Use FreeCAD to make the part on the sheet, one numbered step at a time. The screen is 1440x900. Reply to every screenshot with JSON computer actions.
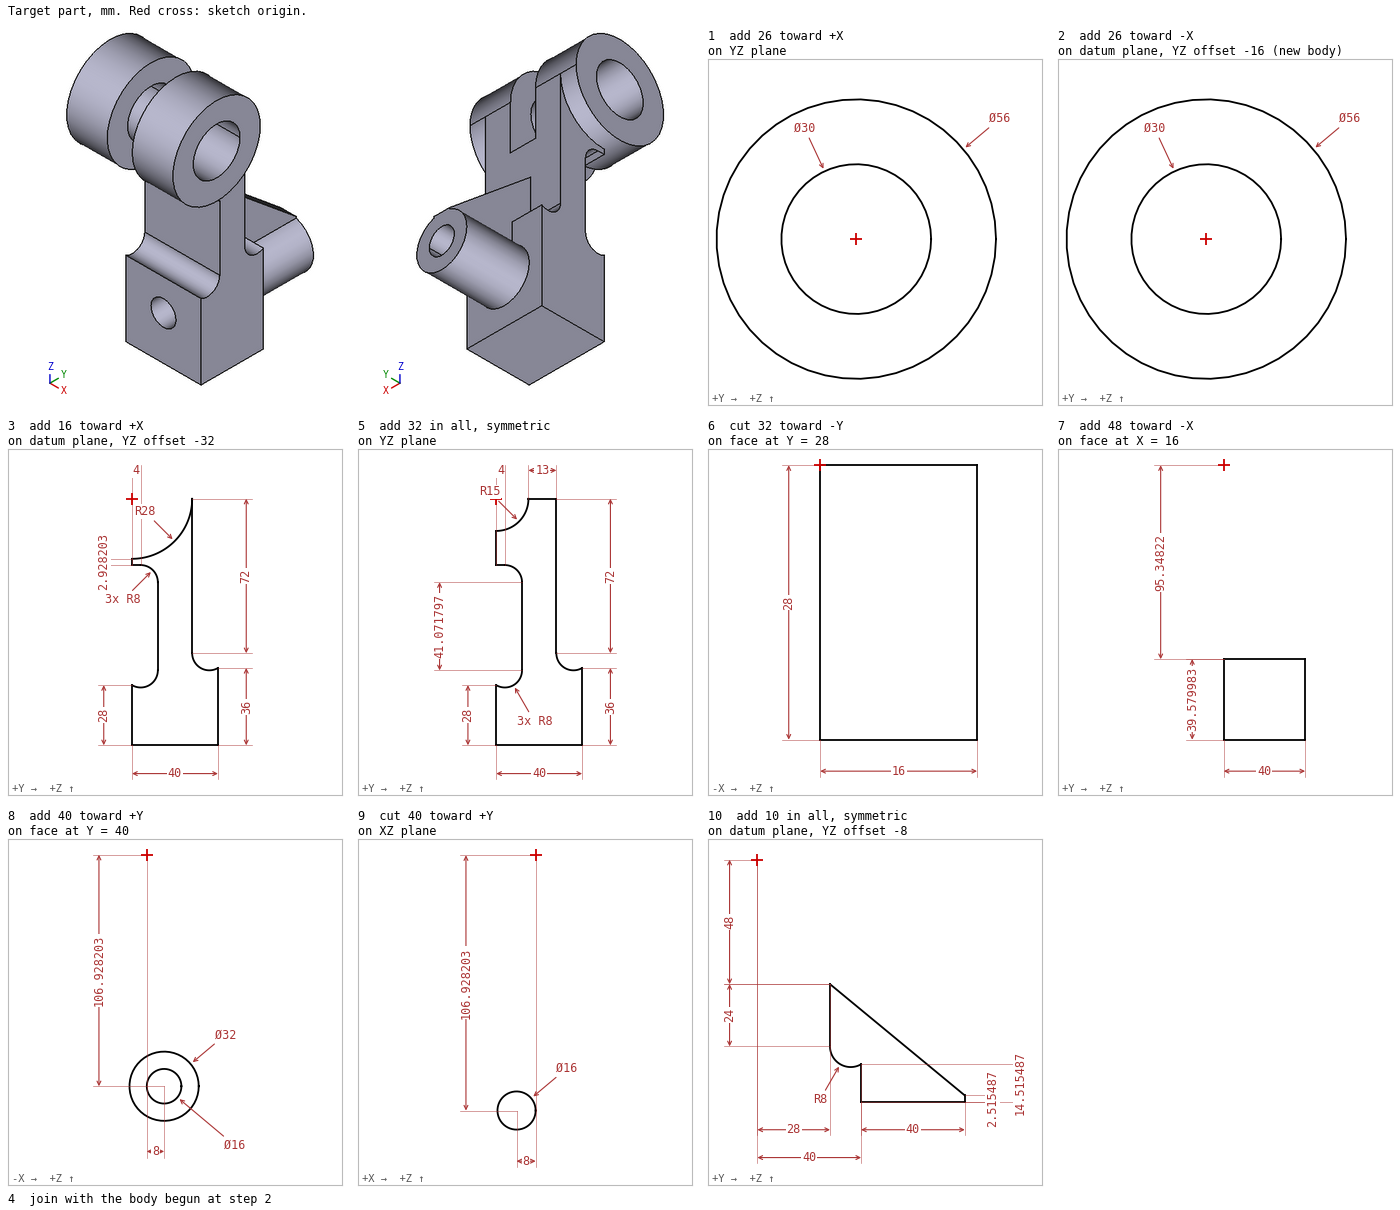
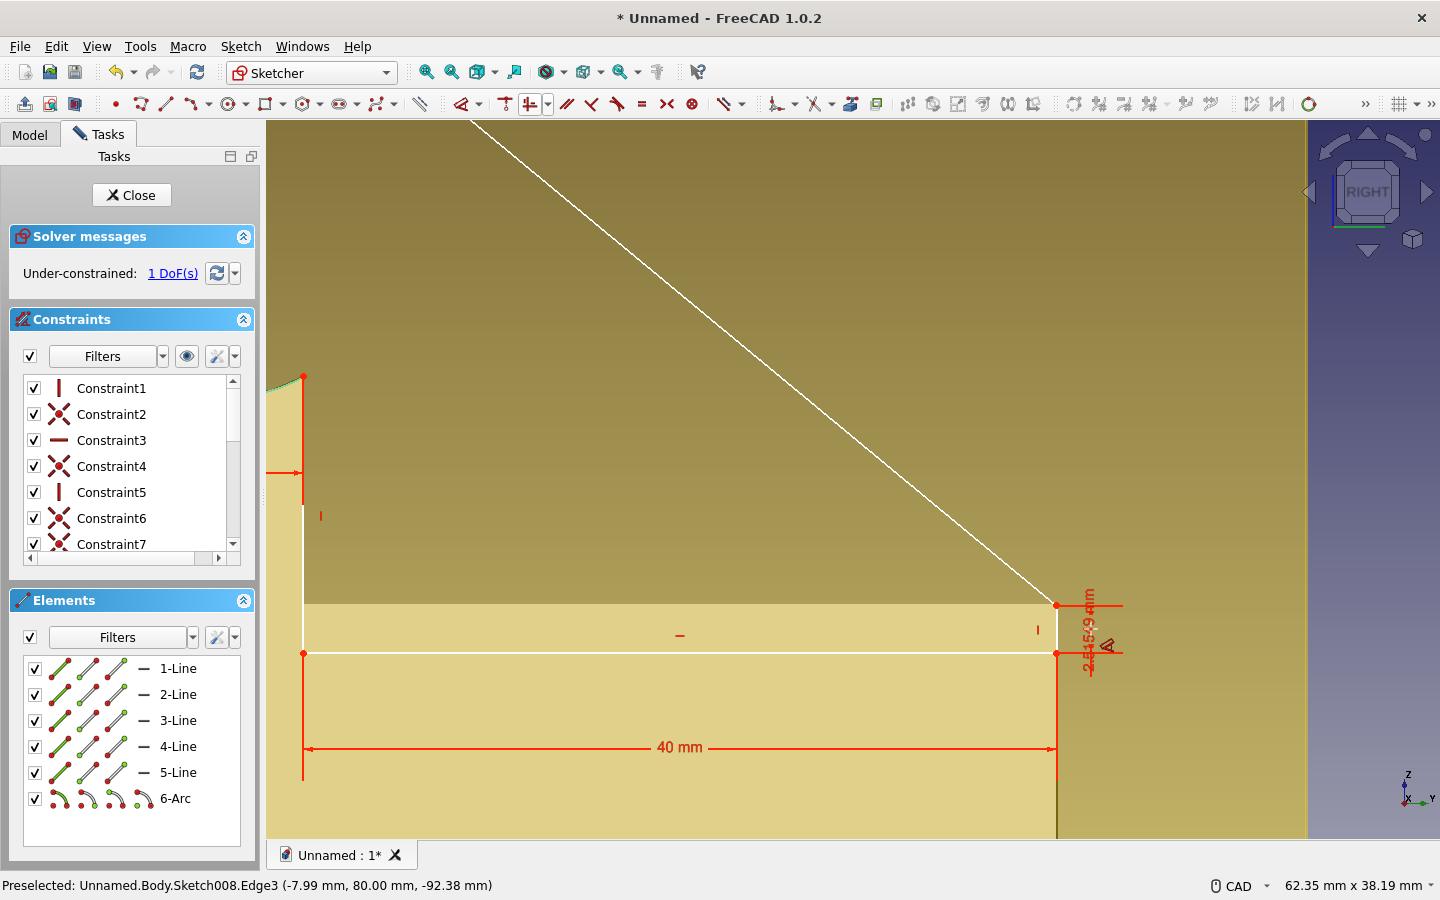
{"action": "scroll", "coordinate": [942, 712], "scroll_direction": "down", "scroll_amount": 7}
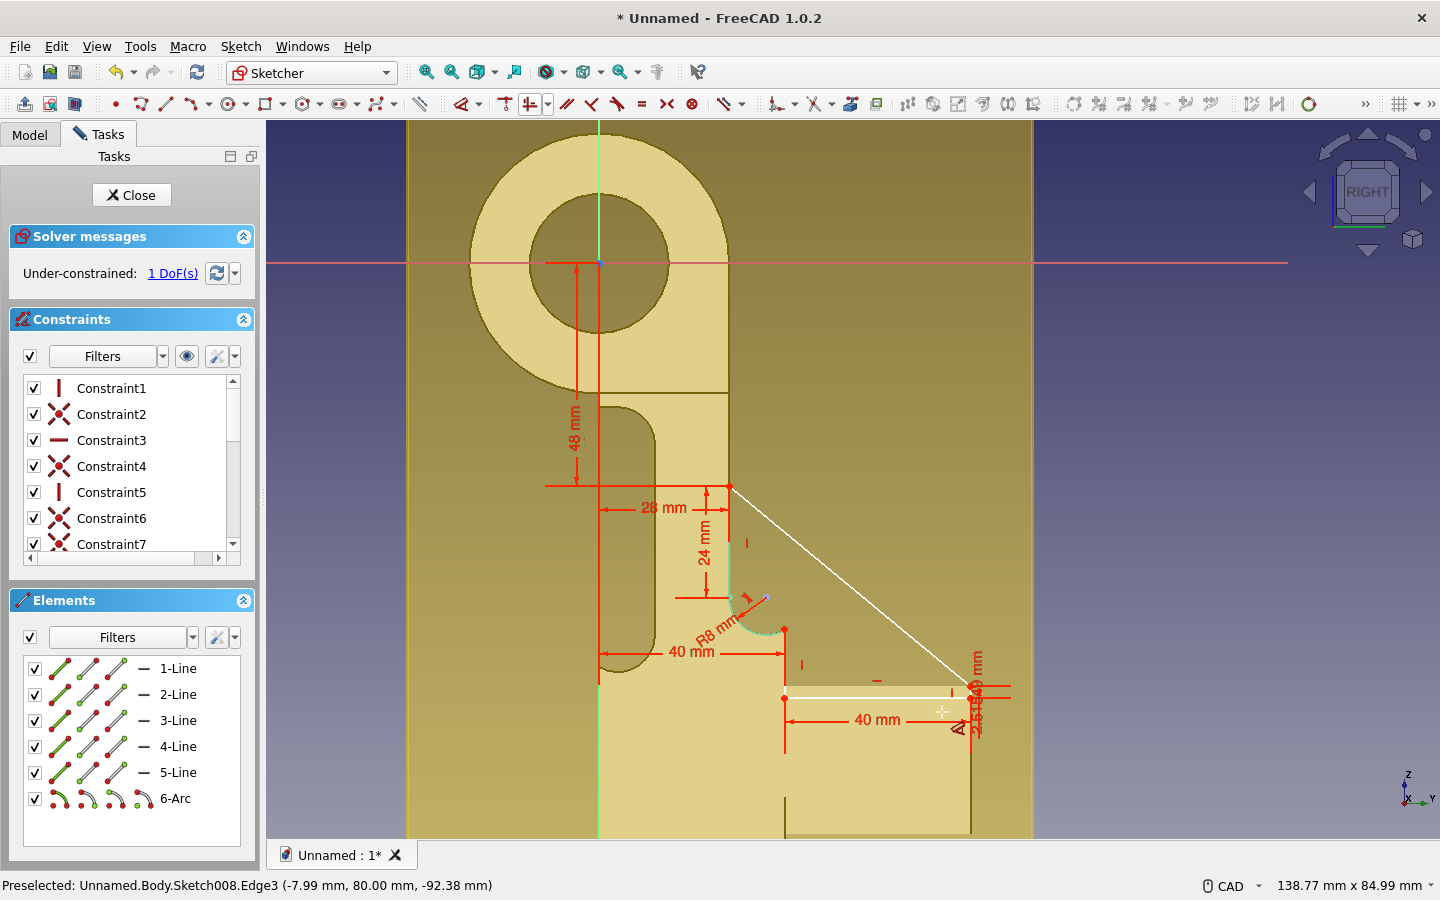
{"action": "left_click", "coordinate": [785, 650]}
{"action": "left_click", "coordinate": [819, 664]}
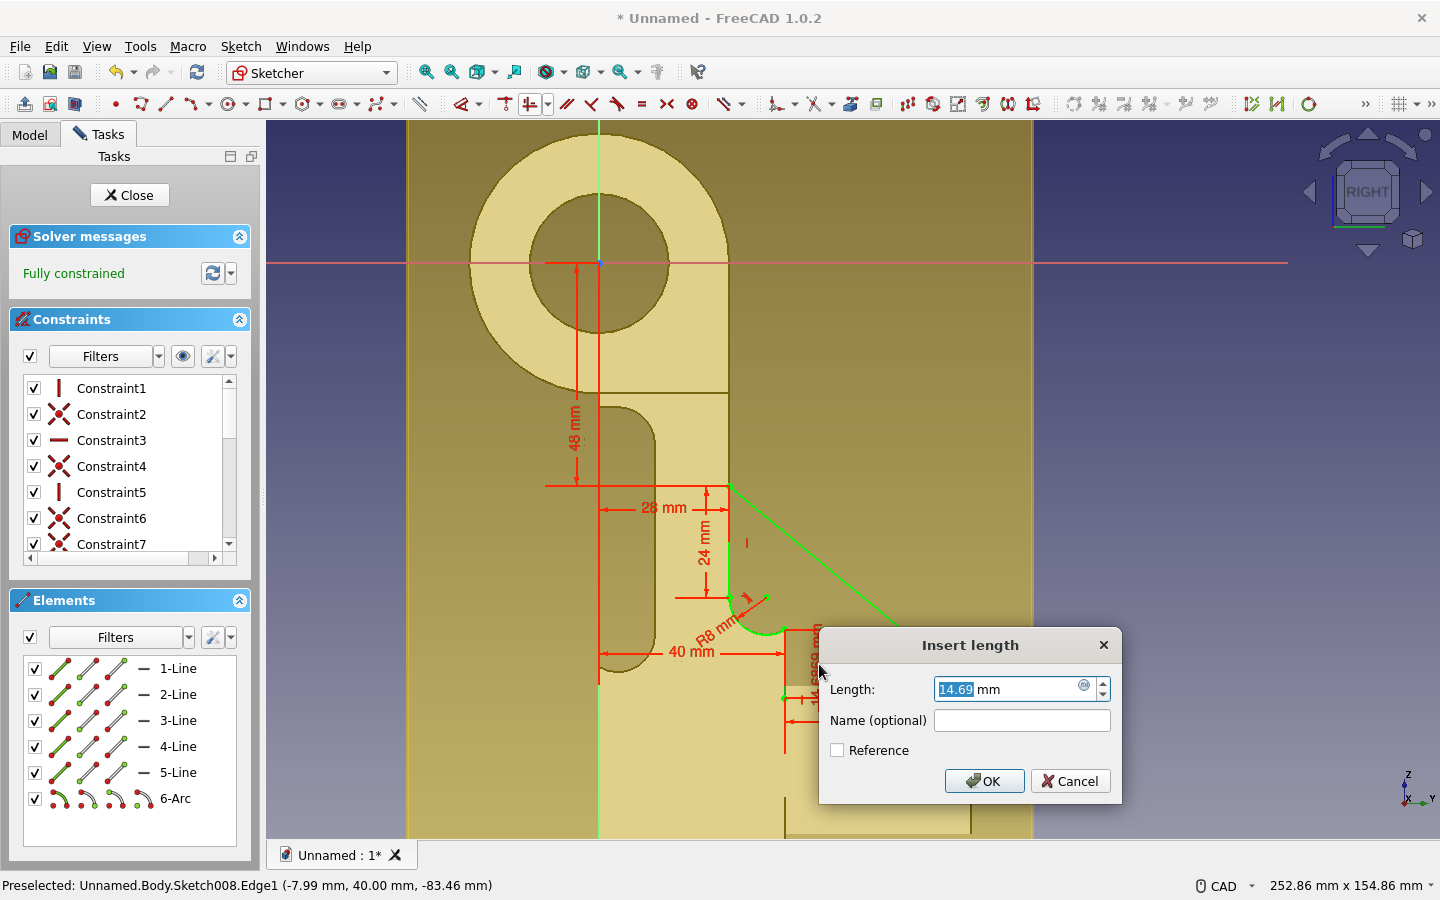
{"action": "type", "text": "14.515487"}
{"action": "key", "text": "Return"}
{"action": "key", "text": "Escape"}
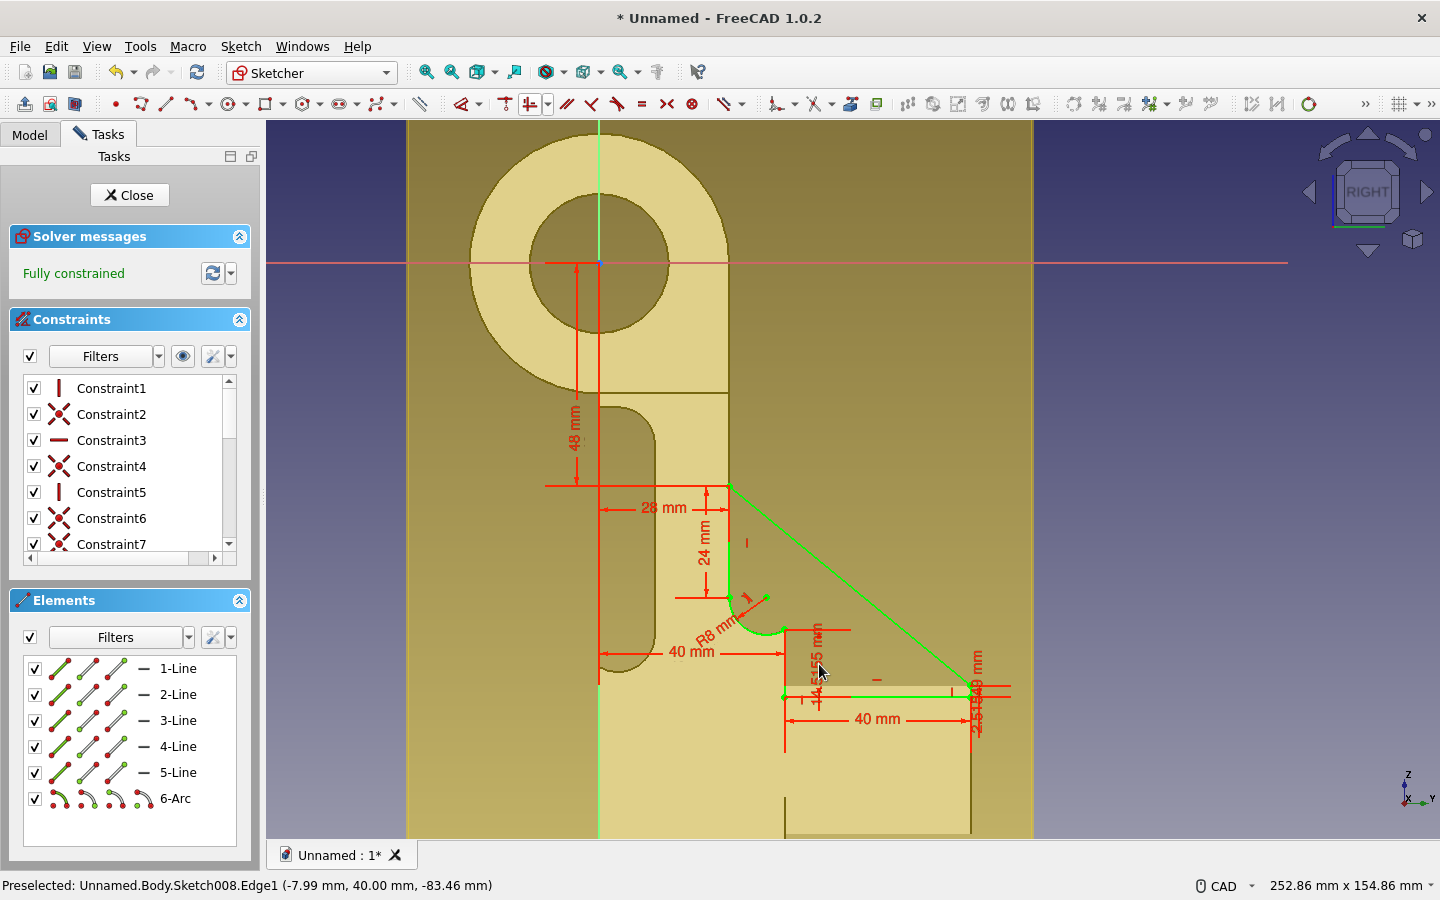
{"action": "left_click", "coordinate": [130, 195]}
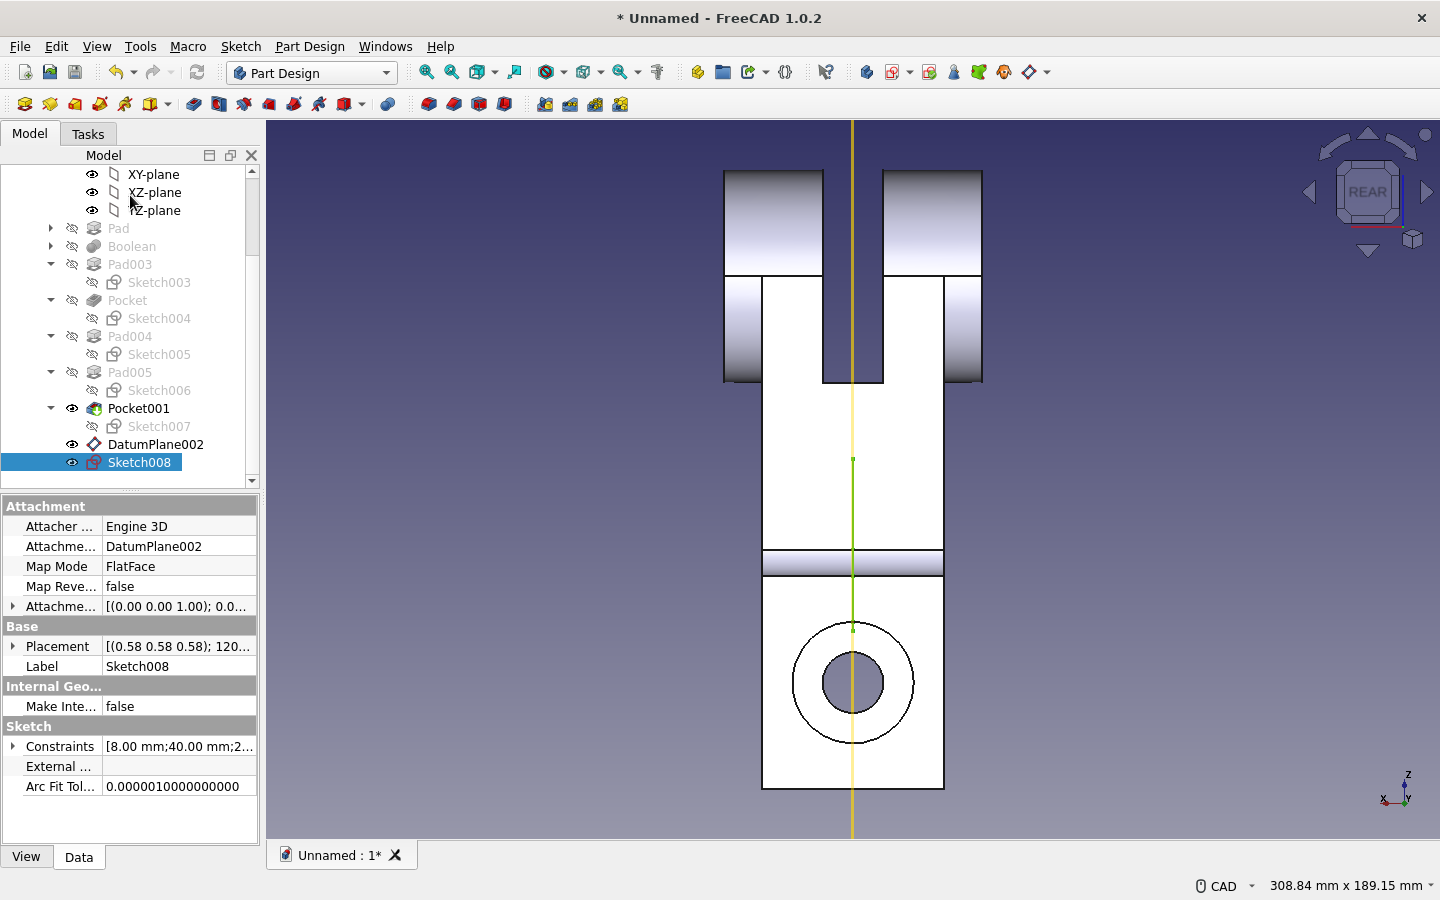
{"action": "left_click", "coordinate": [25, 104]}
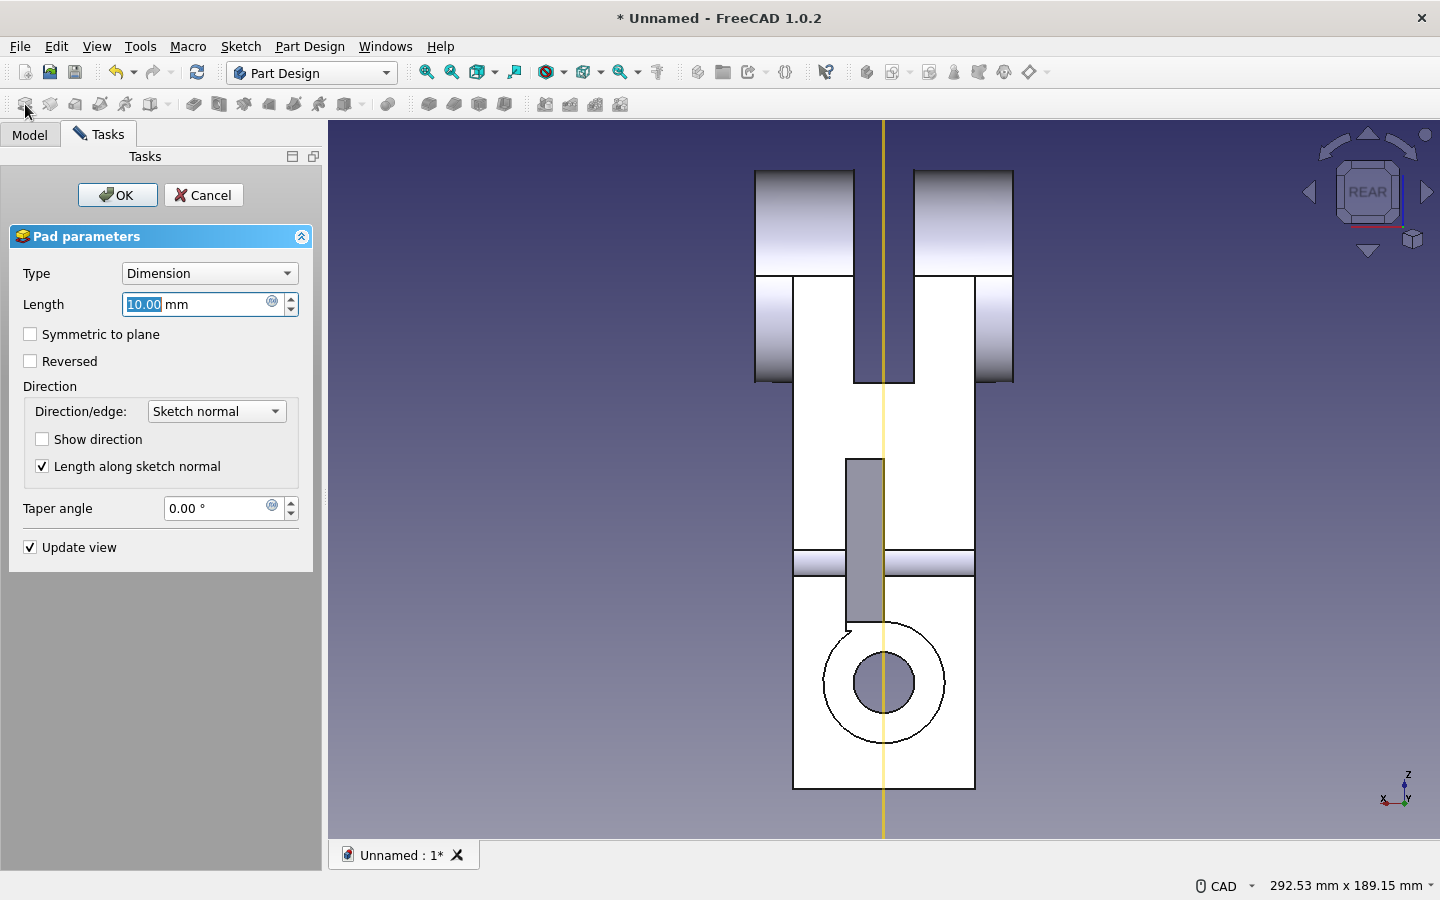
{"action": "type", "text": "10"}
{"action": "key", "text": "Tab"}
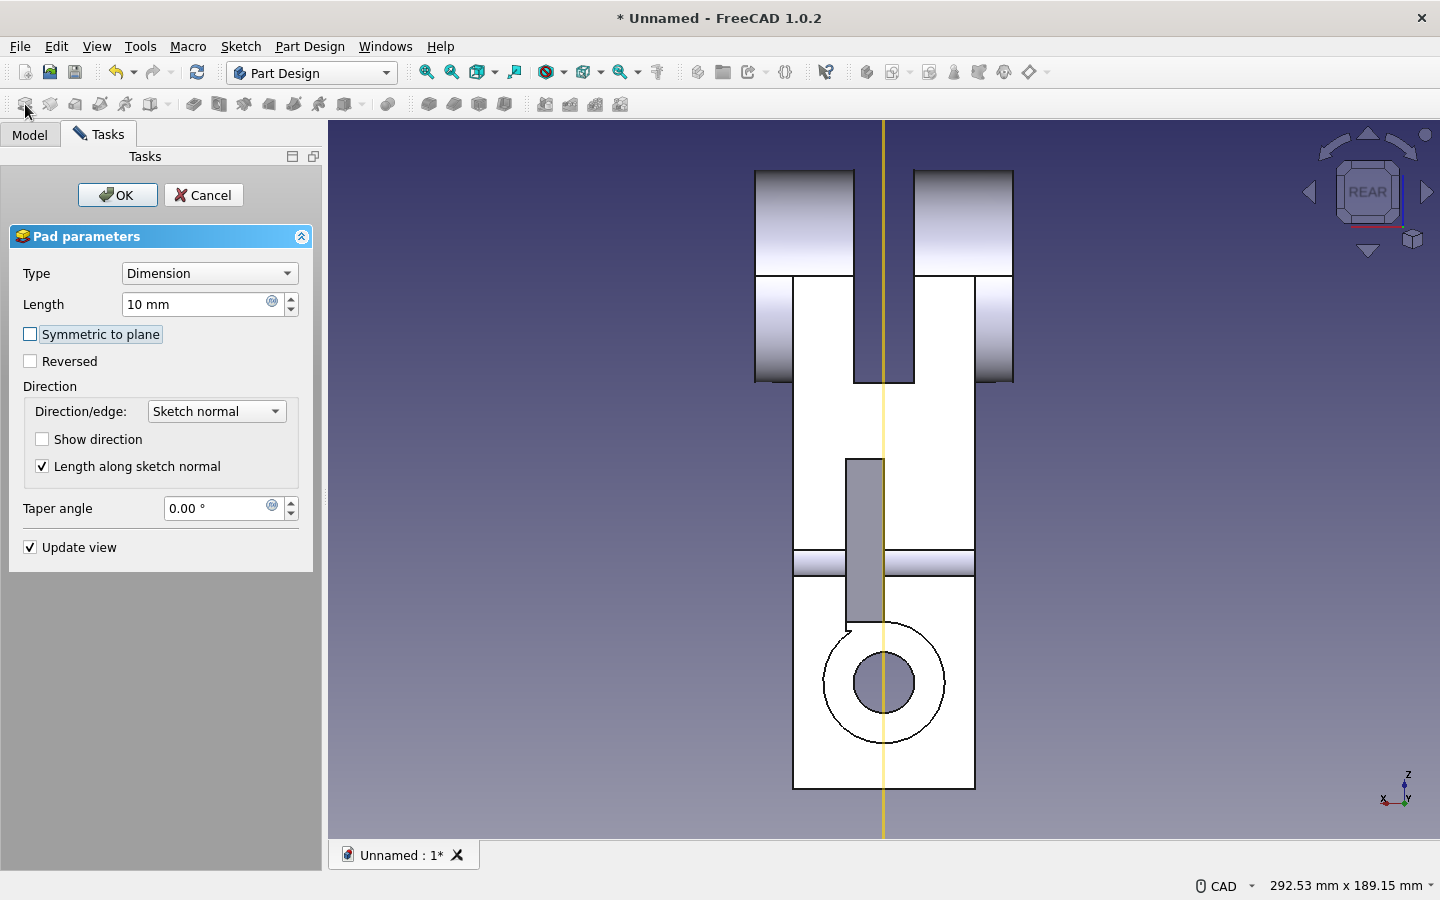
{"action": "left_click", "coordinate": [31, 334]}